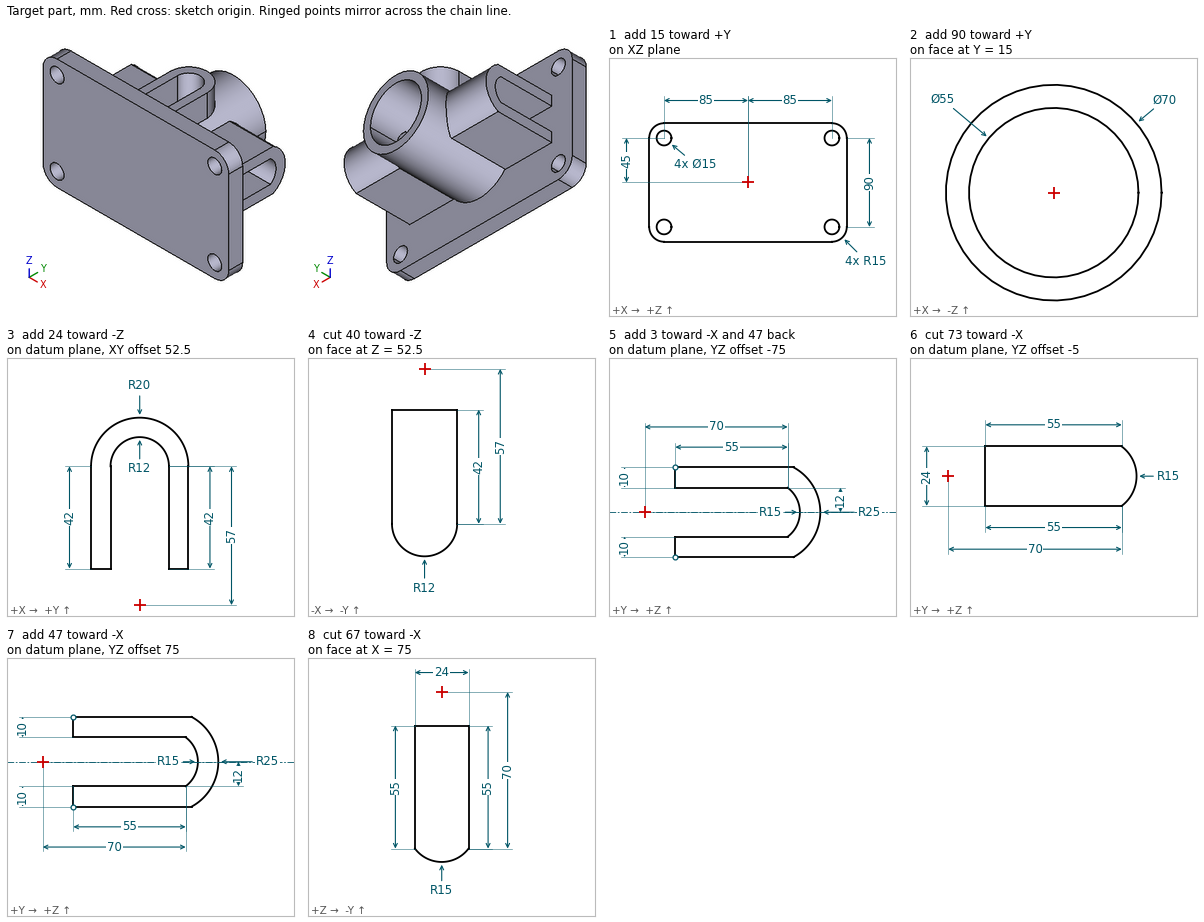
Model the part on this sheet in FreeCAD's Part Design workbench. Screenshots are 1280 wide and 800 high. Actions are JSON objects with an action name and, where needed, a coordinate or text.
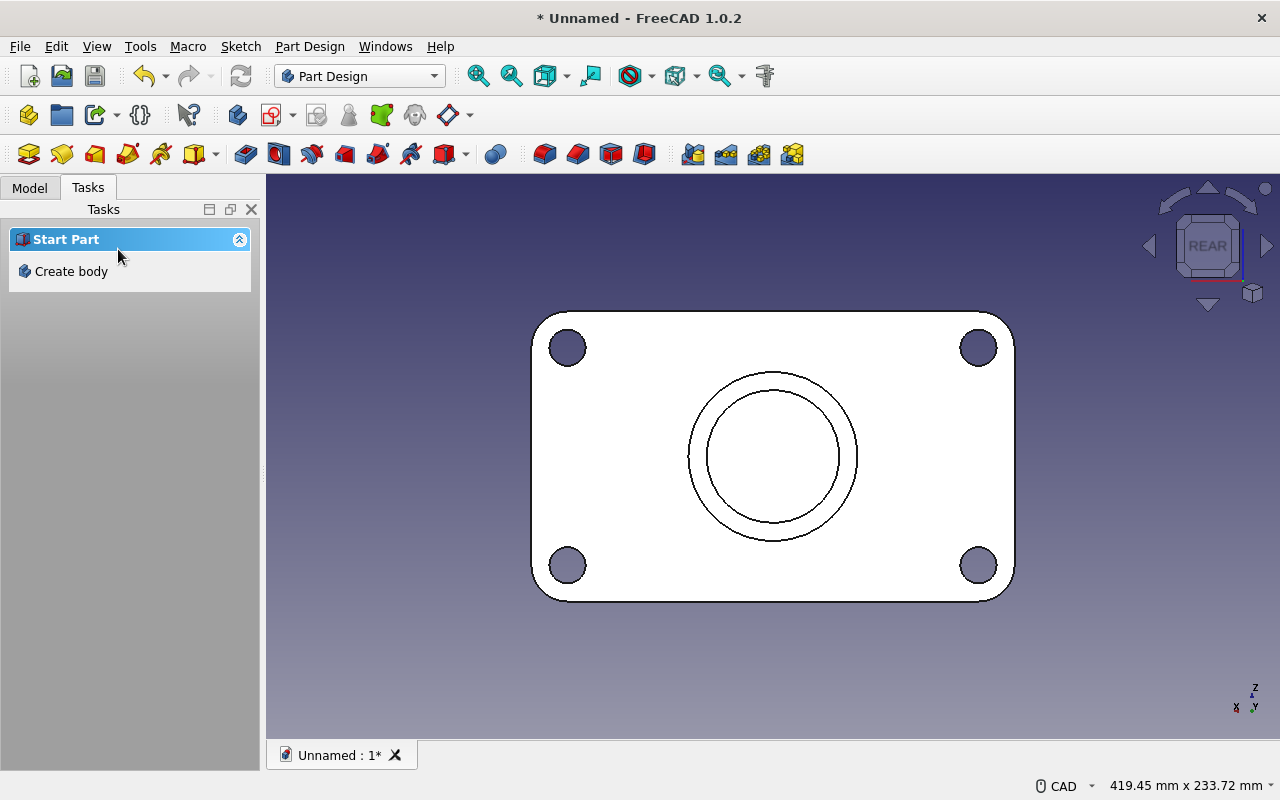
{"action": "left_click", "coordinate": [30, 188]}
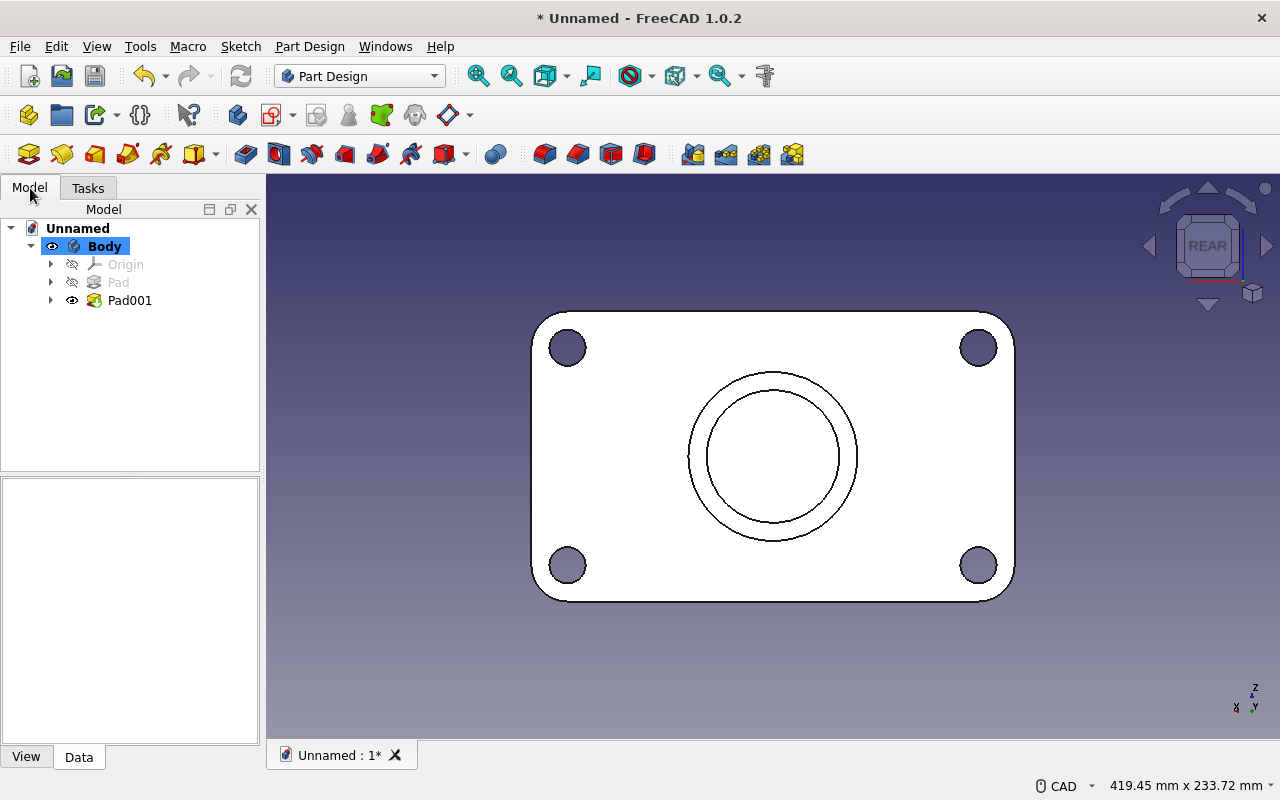
{"action": "left_click", "coordinate": [51, 264]}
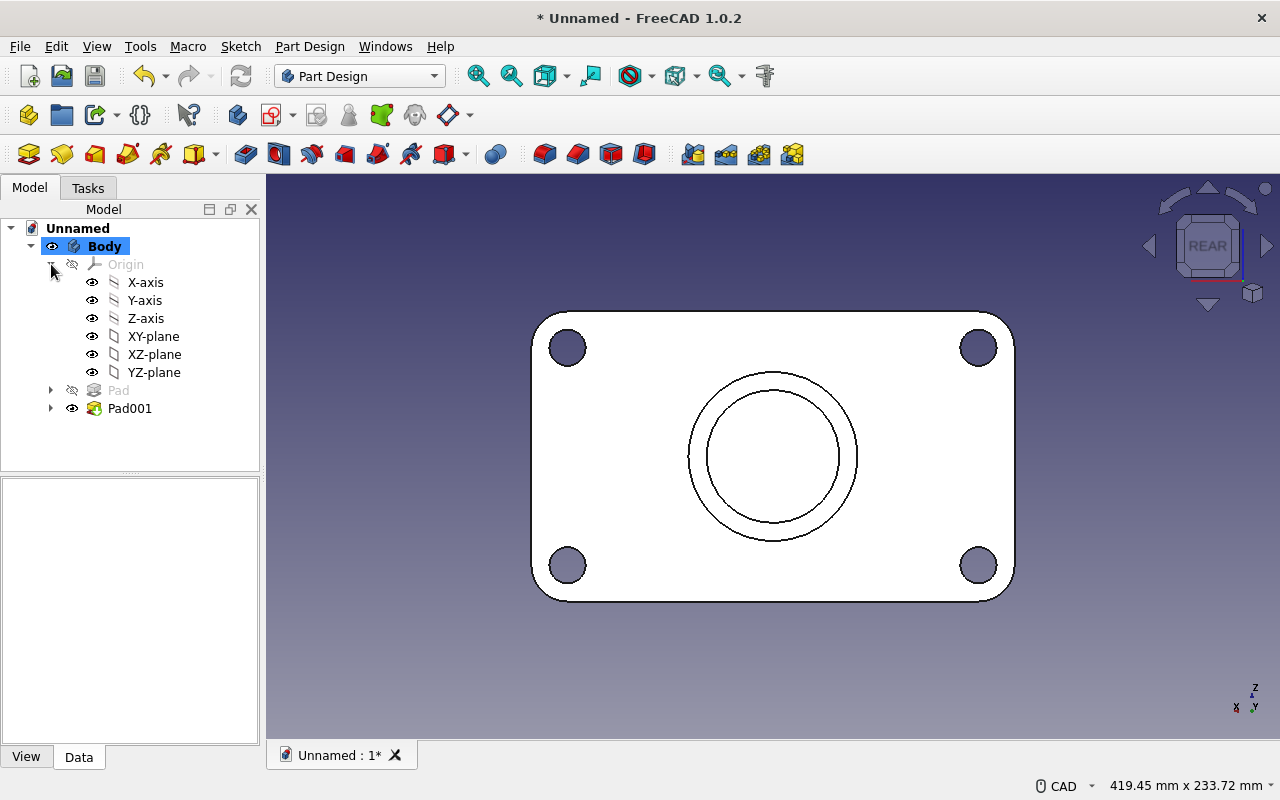
{"action": "left_click", "coordinate": [137, 336]}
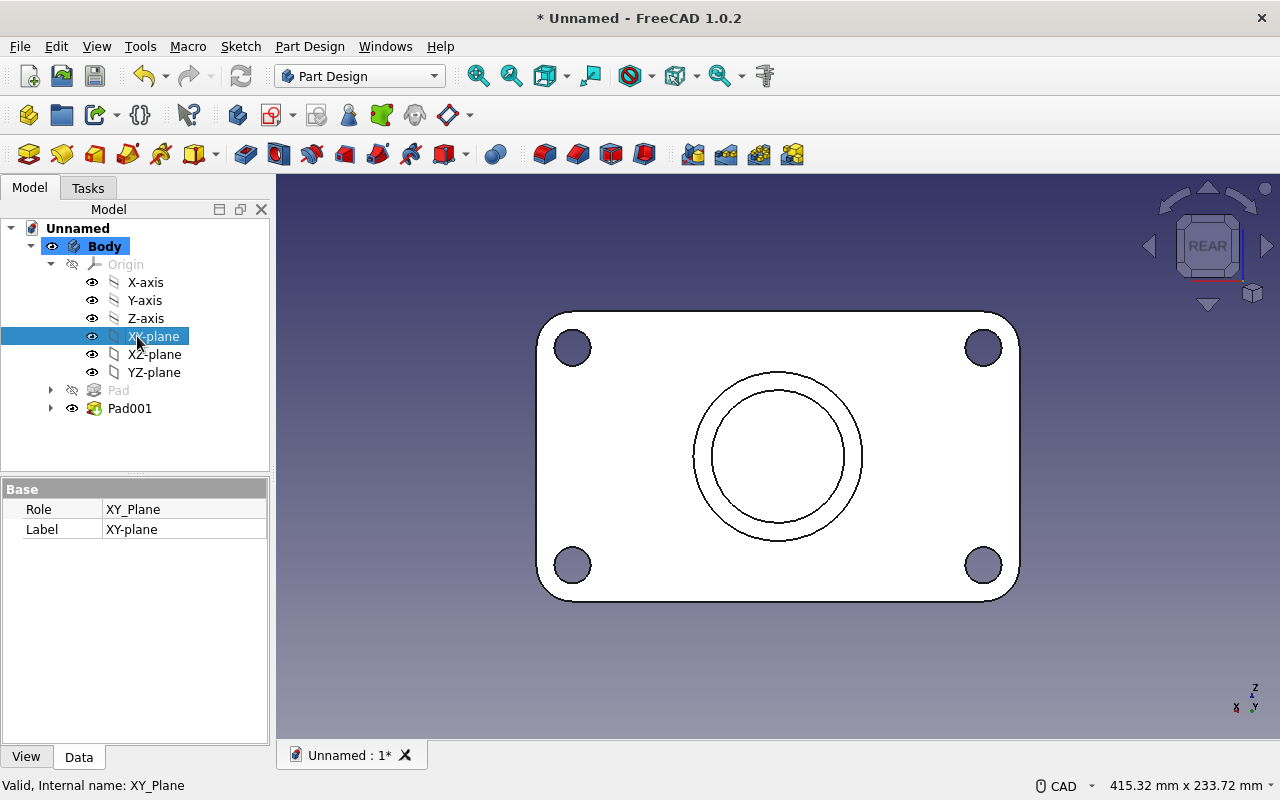
{"action": "left_click", "coordinate": [448, 116]}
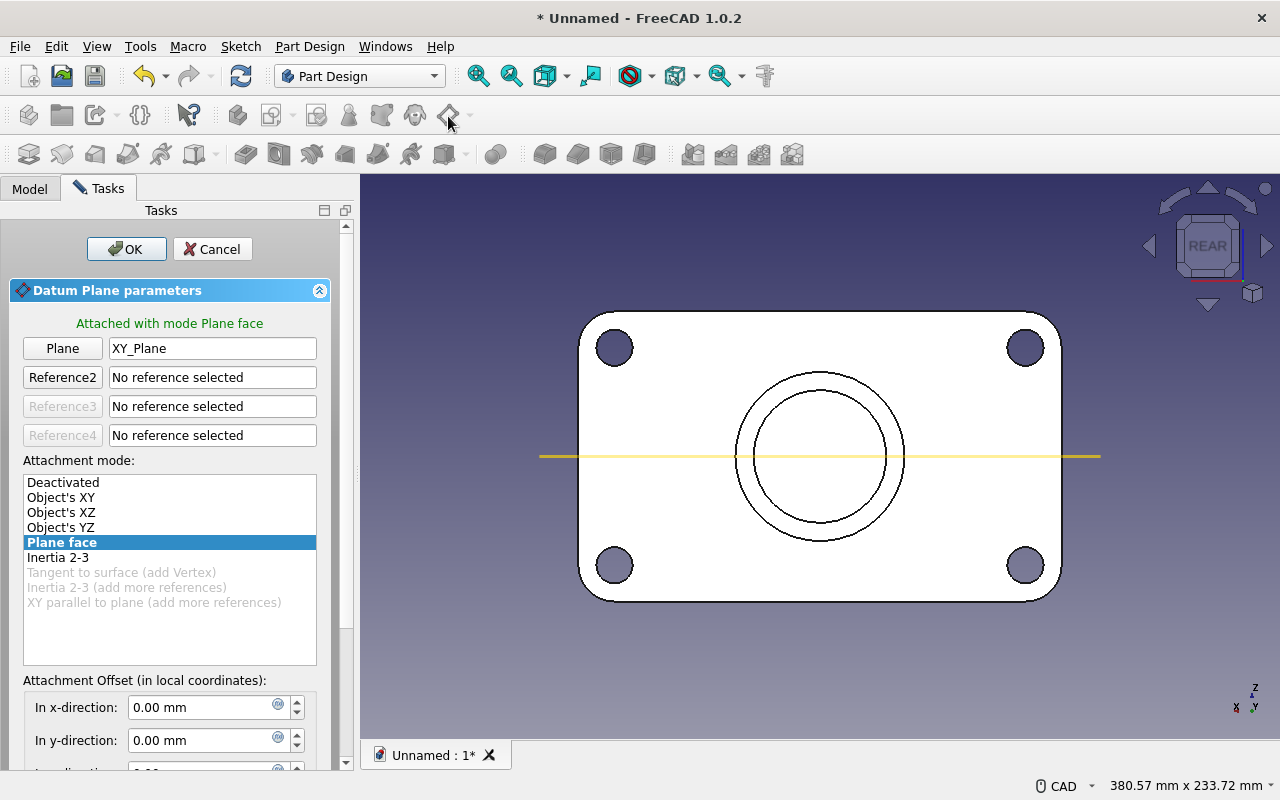
{"action": "scroll", "coordinate": [346, 495], "scroll_direction": "down", "scroll_amount": 2}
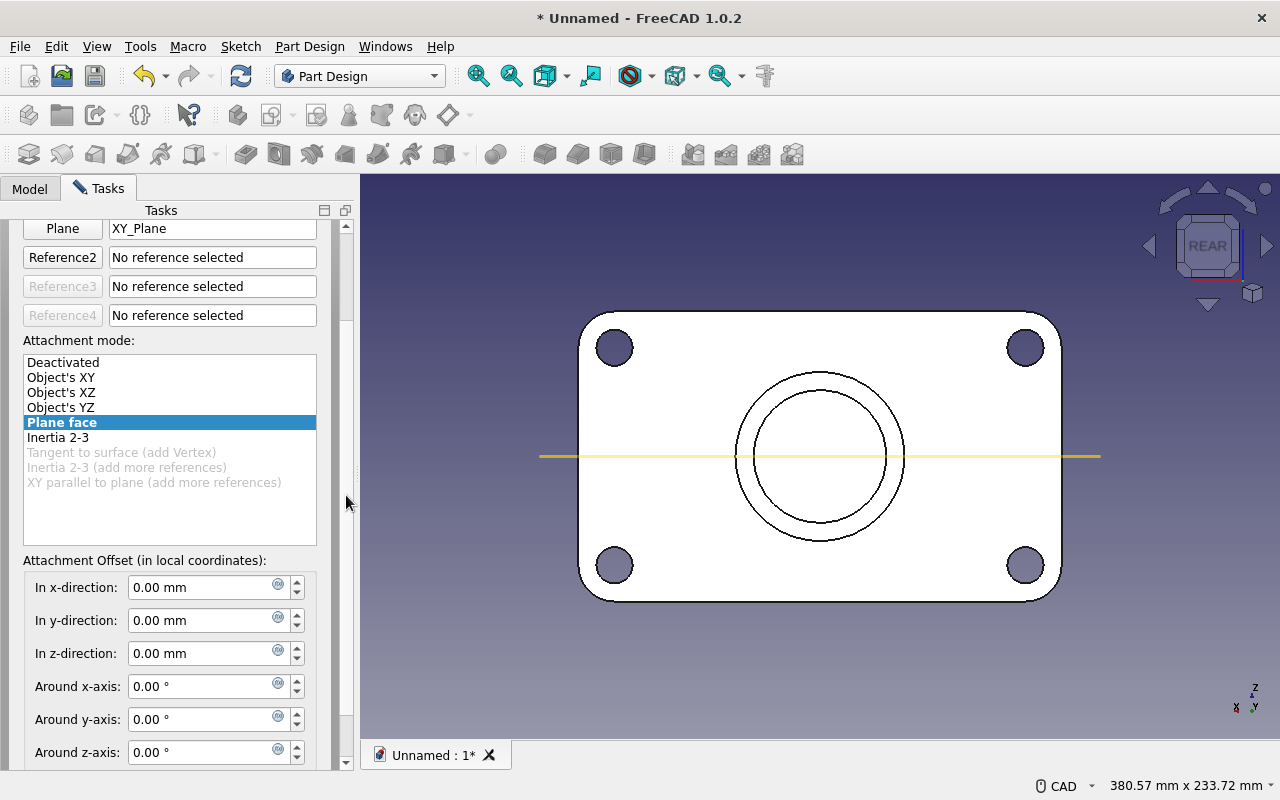
{"action": "triple_click", "coordinate": [210, 654]}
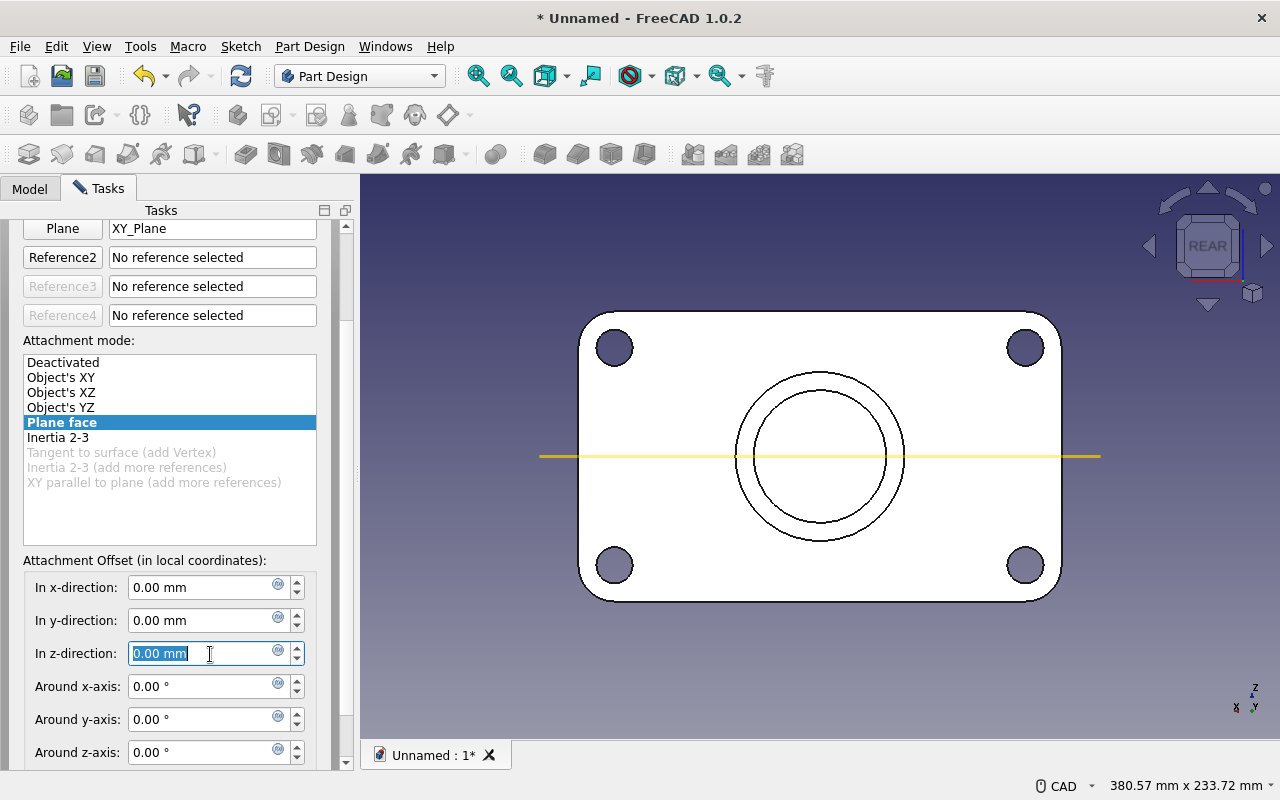
{"action": "type", "text": "52.5"}
{"action": "key", "text": "Tab"}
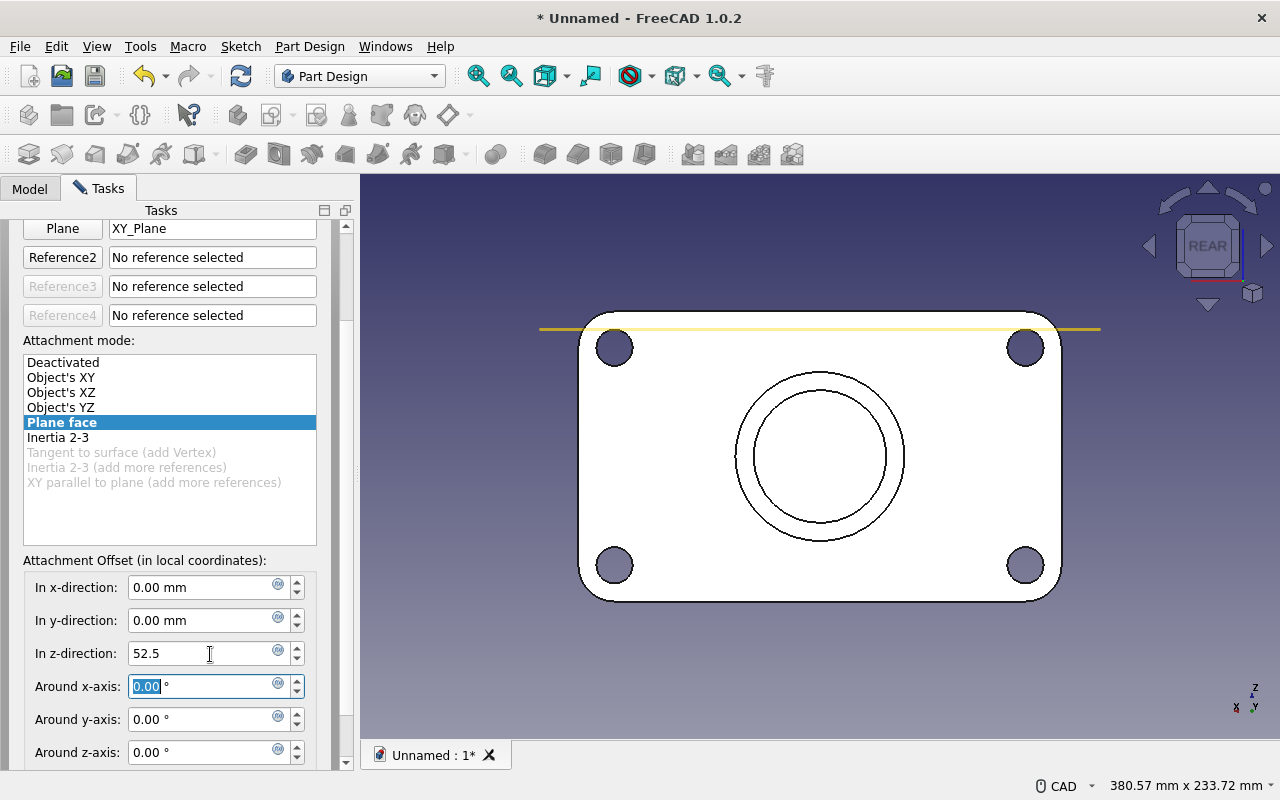
{"action": "scroll", "coordinate": [346, 495], "scroll_direction": "up", "scroll_amount": 3}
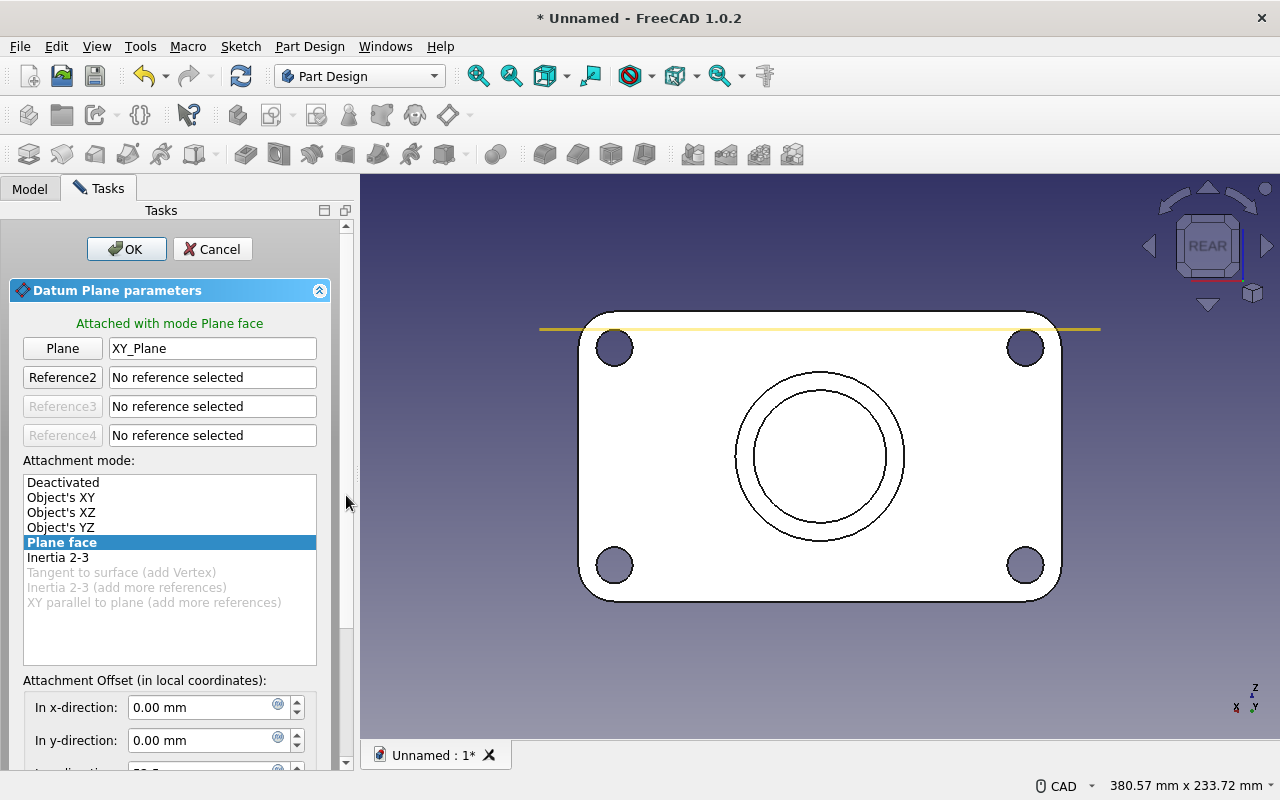
{"action": "left_click", "coordinate": [127, 249]}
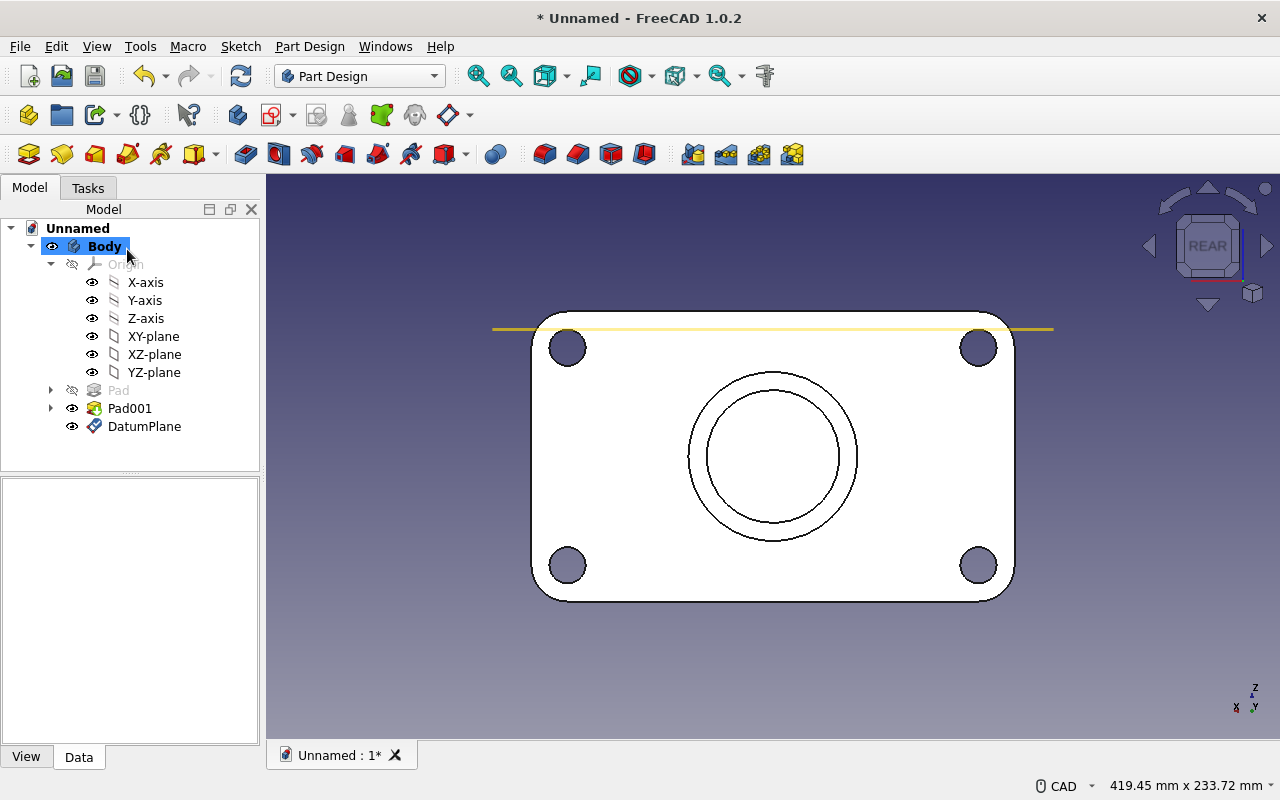
{"action": "left_click", "coordinate": [117, 426]}